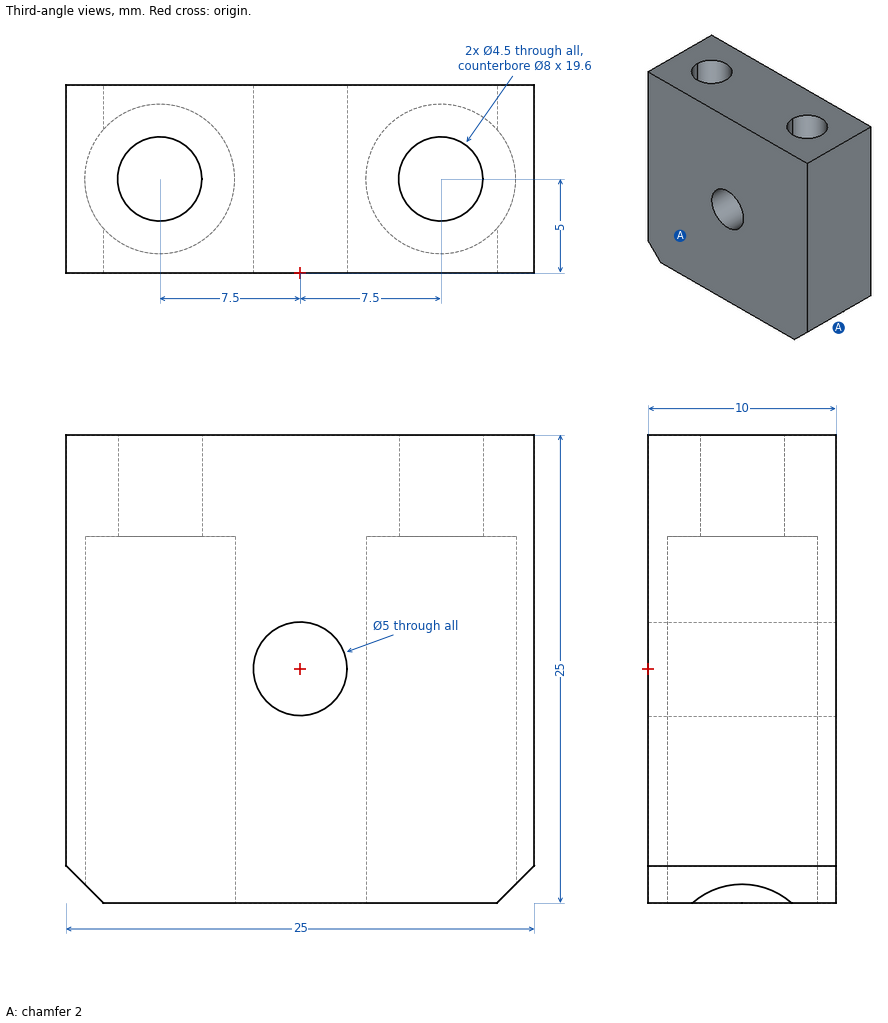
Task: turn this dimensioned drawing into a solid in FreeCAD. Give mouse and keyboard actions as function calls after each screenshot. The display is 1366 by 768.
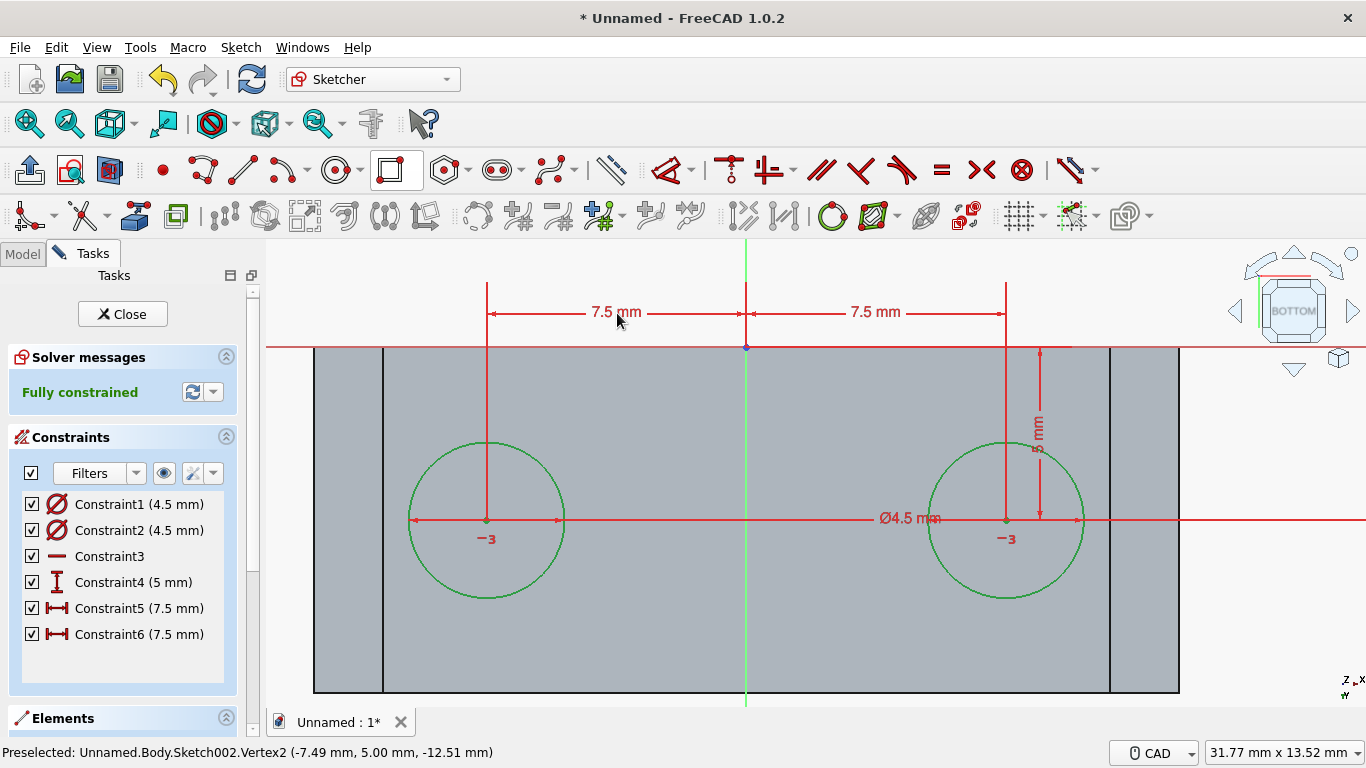
click(123, 314)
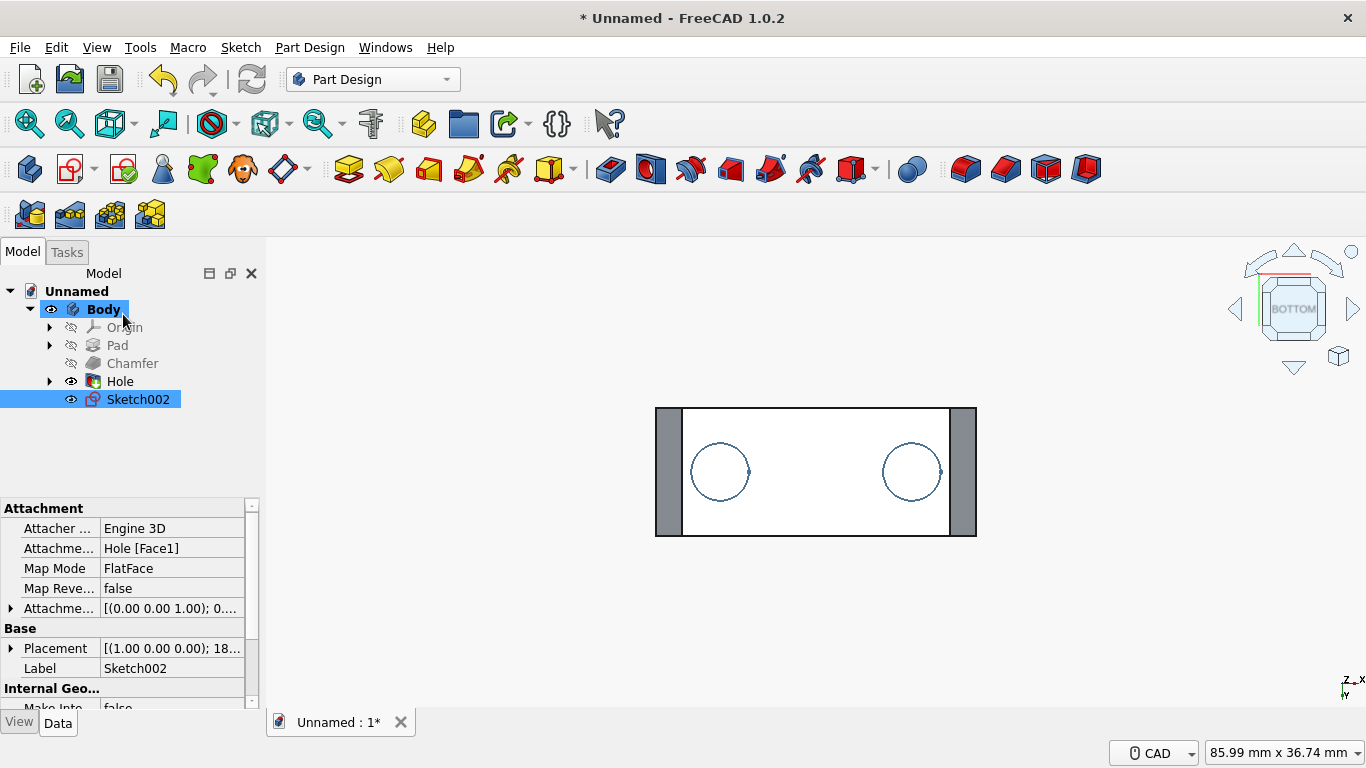
click(652, 170)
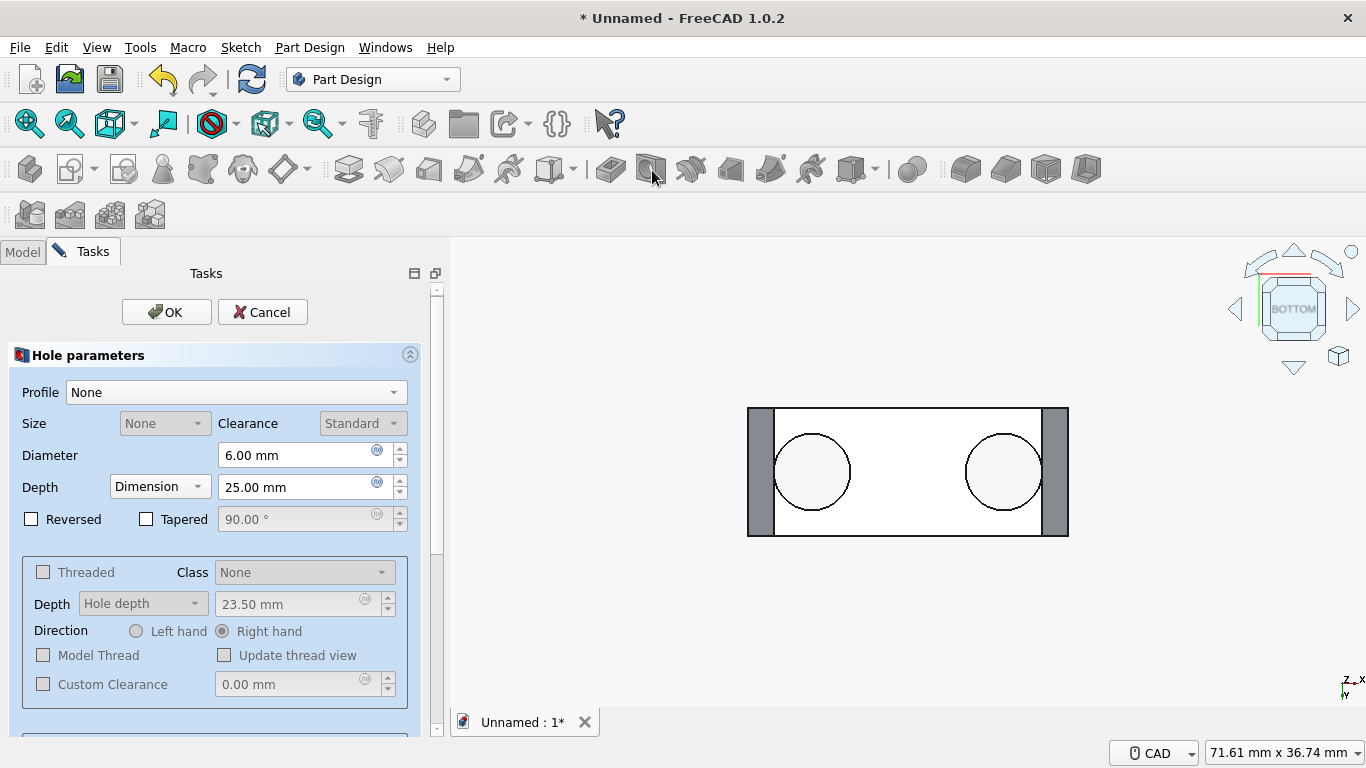
triple_click(305, 455)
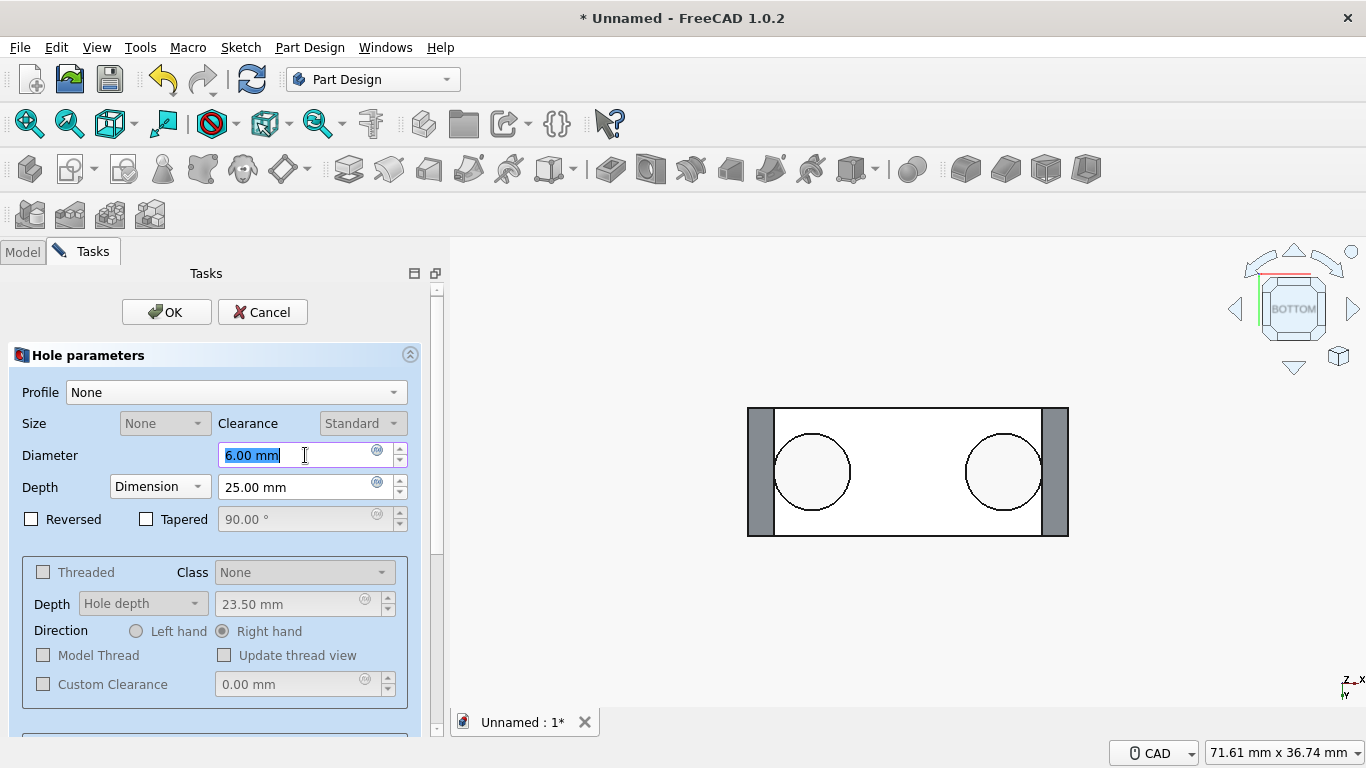
text(4.5)
key(Tab)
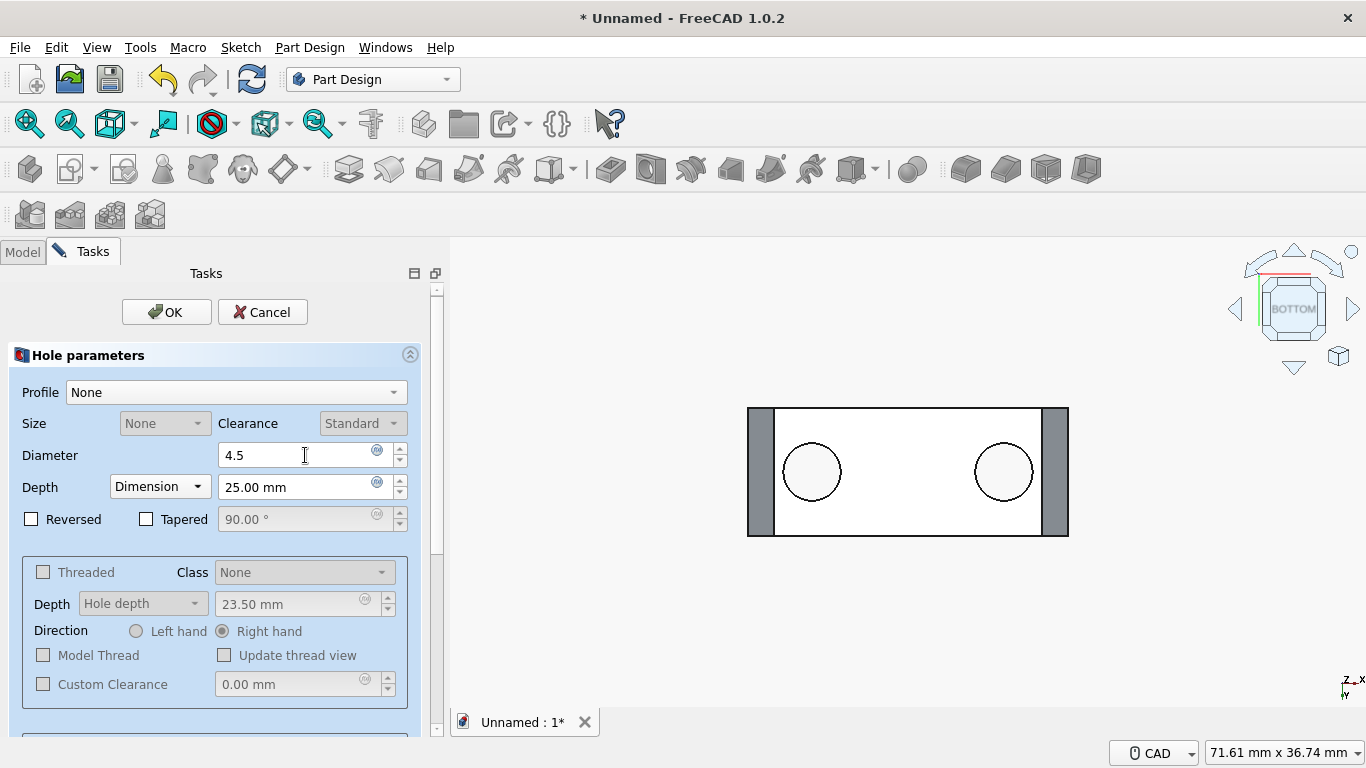
click(161, 486)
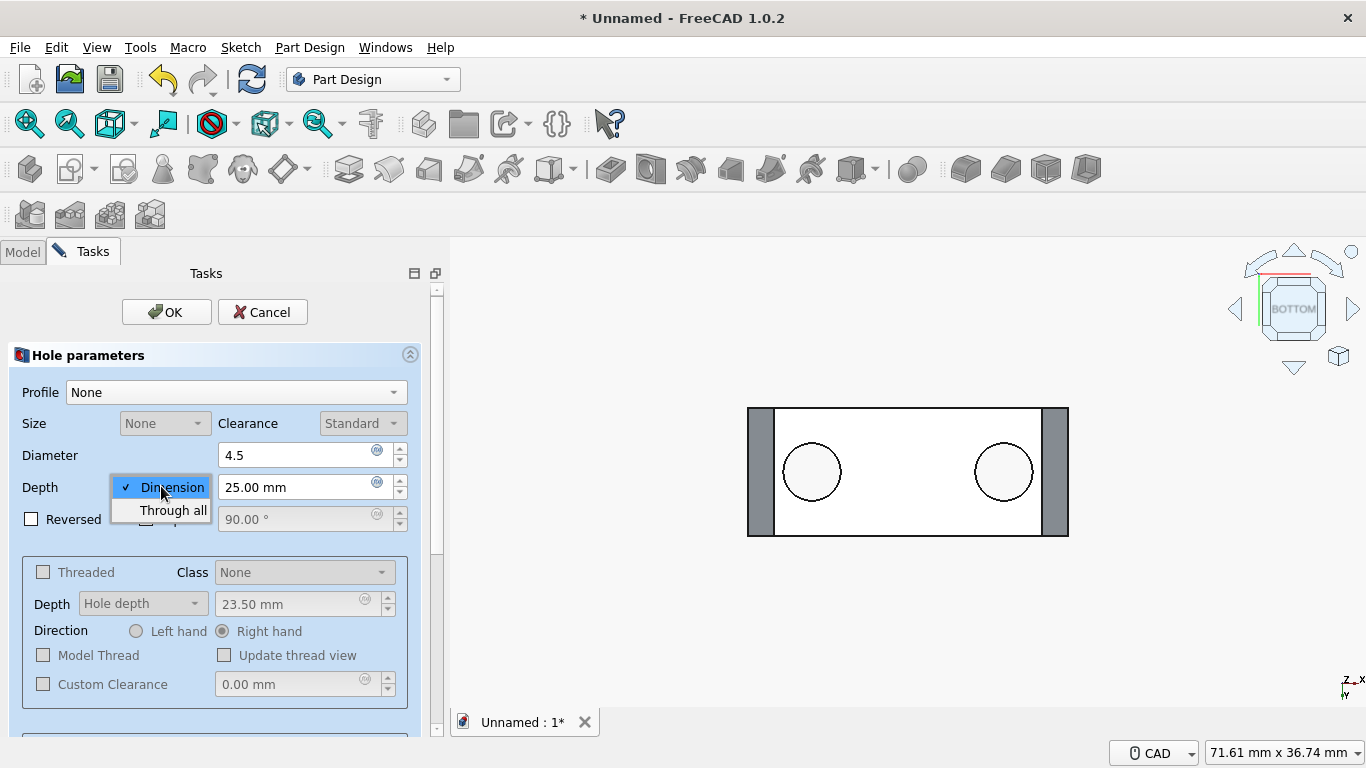
click(160, 510)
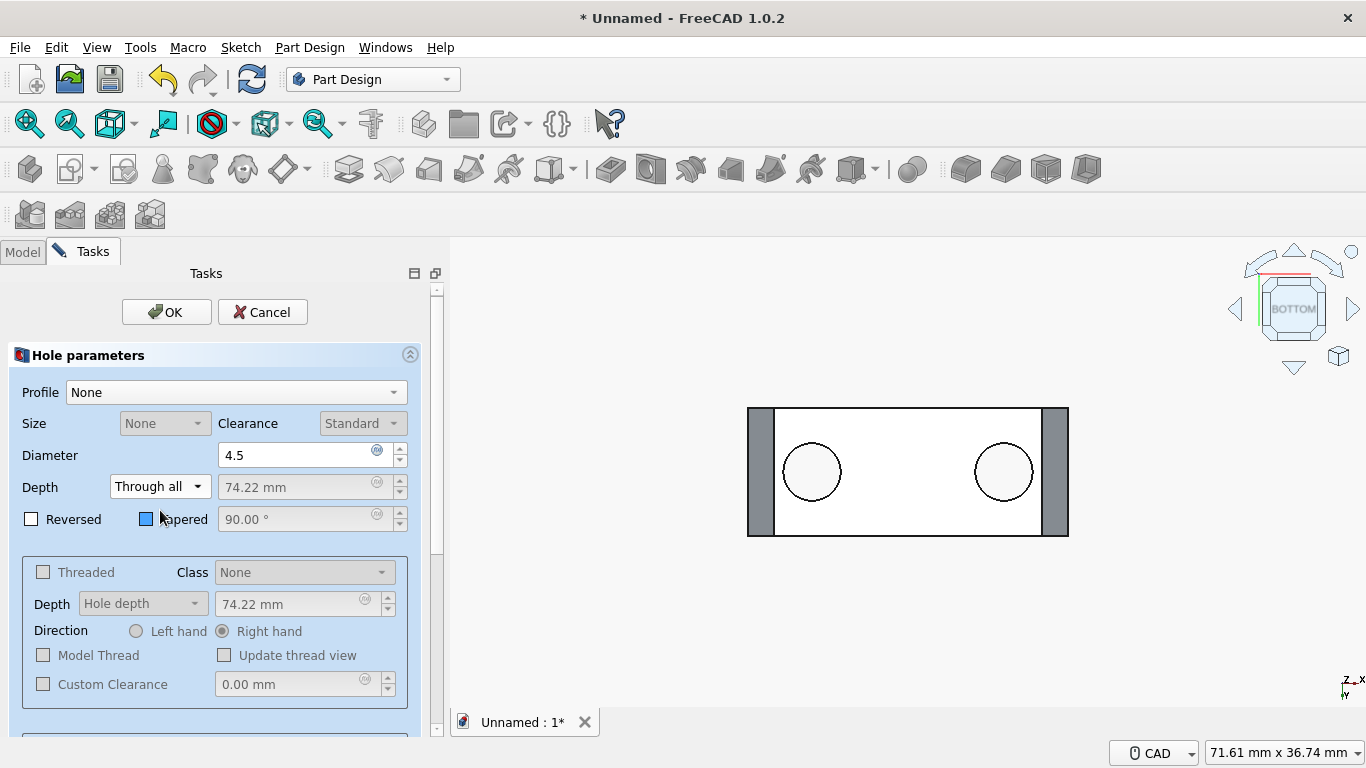
scroll(437, 510, down, 2)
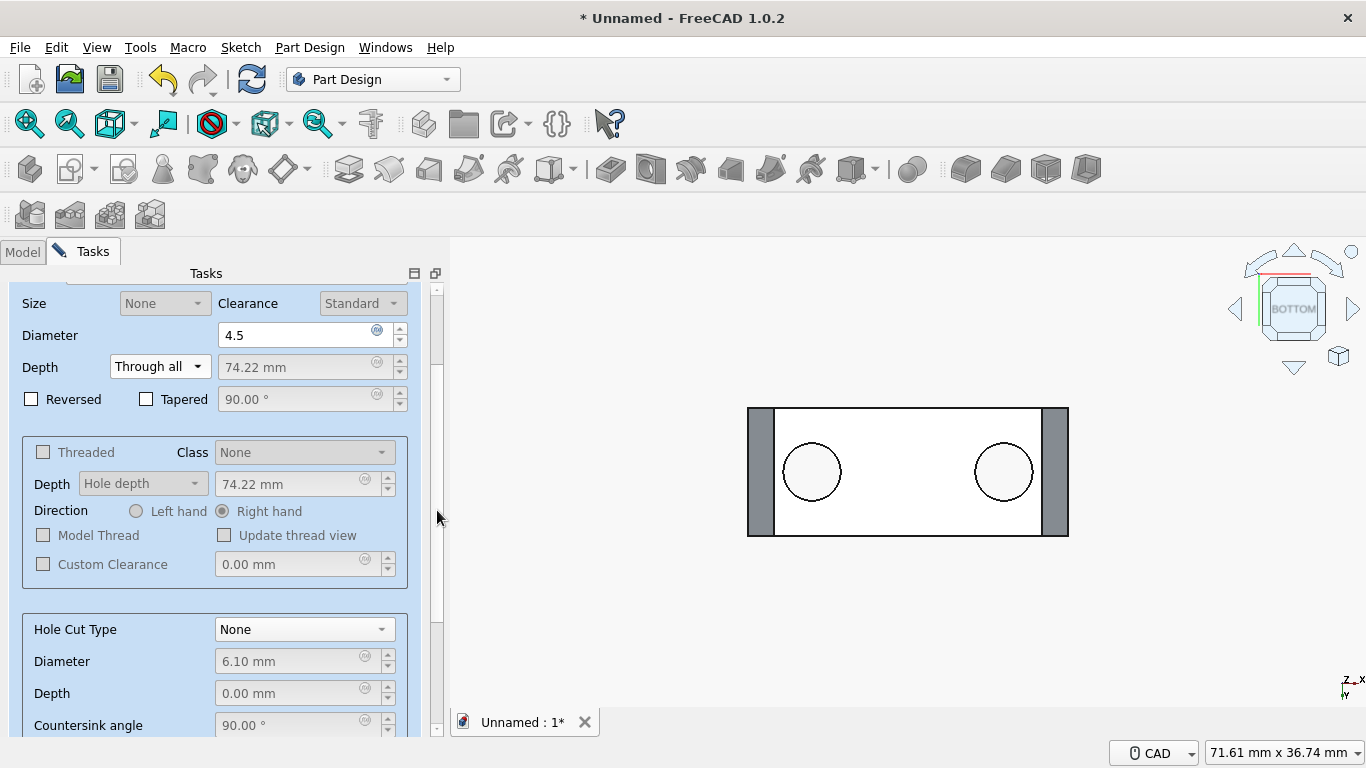
click(306, 630)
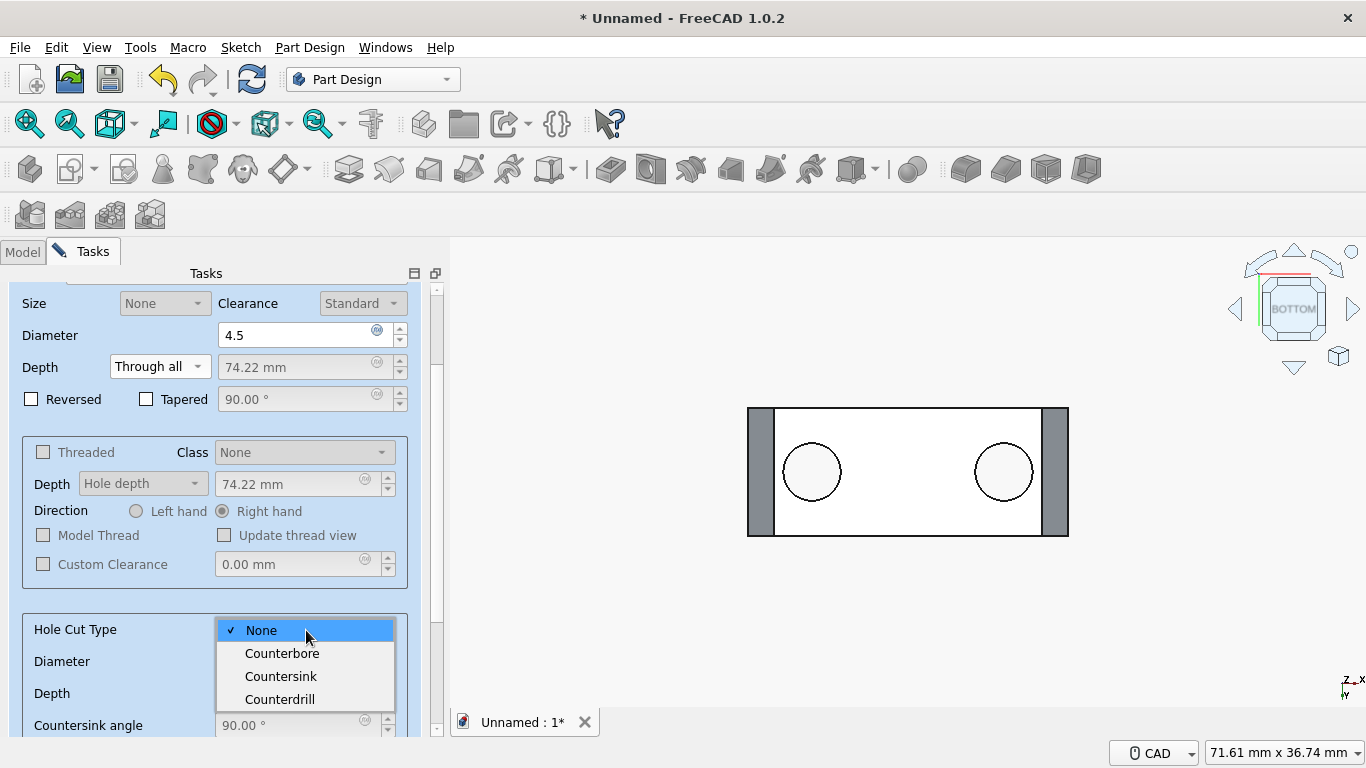
click(304, 654)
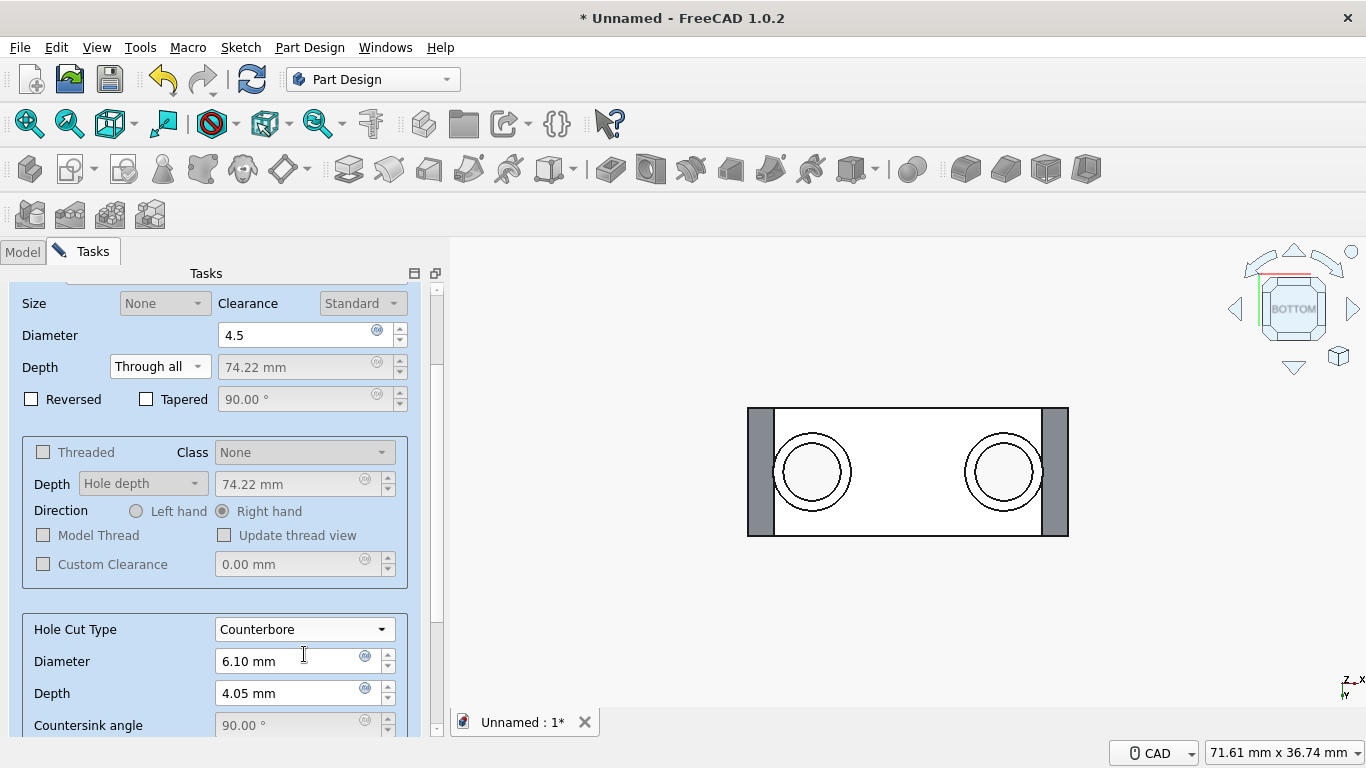
triple_click(298, 661)